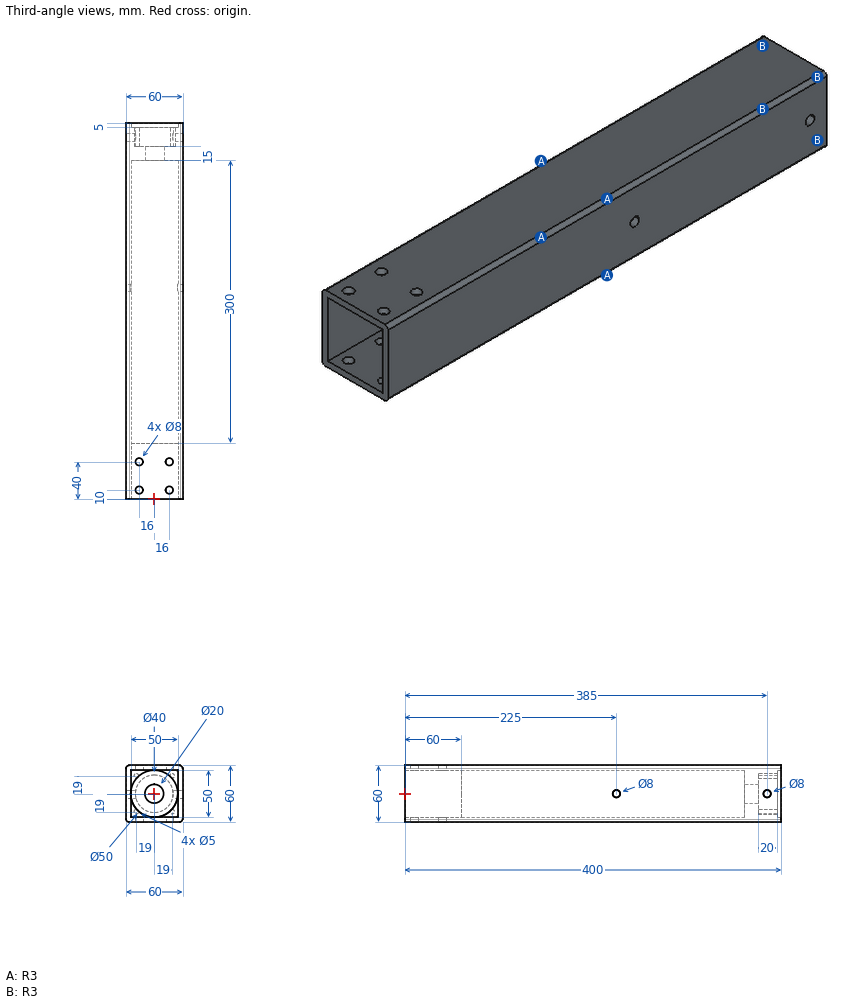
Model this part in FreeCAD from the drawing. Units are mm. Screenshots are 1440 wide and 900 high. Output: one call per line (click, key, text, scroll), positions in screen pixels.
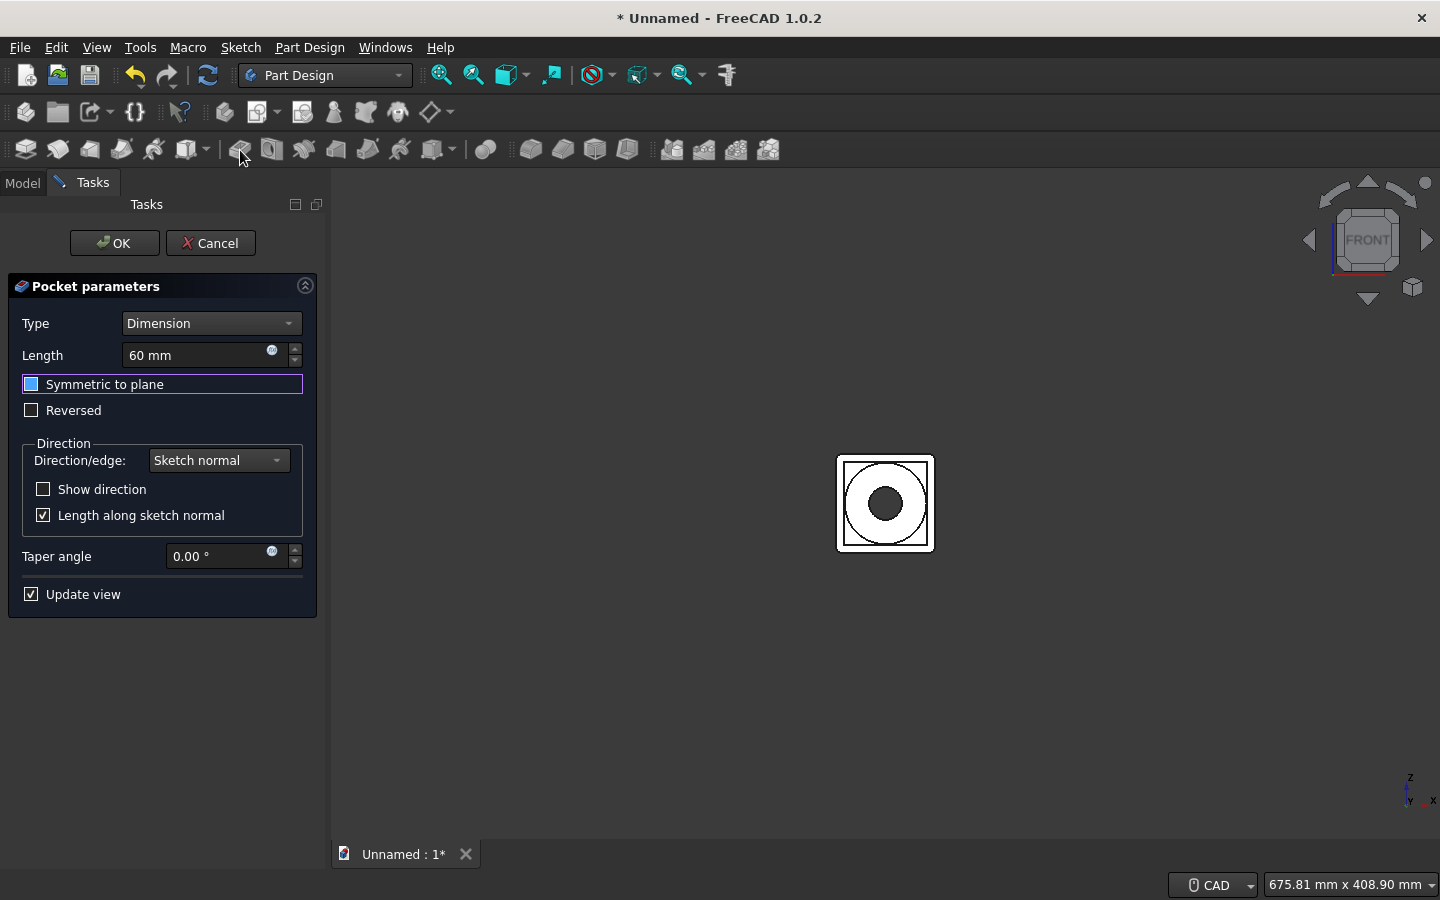
click(30, 384)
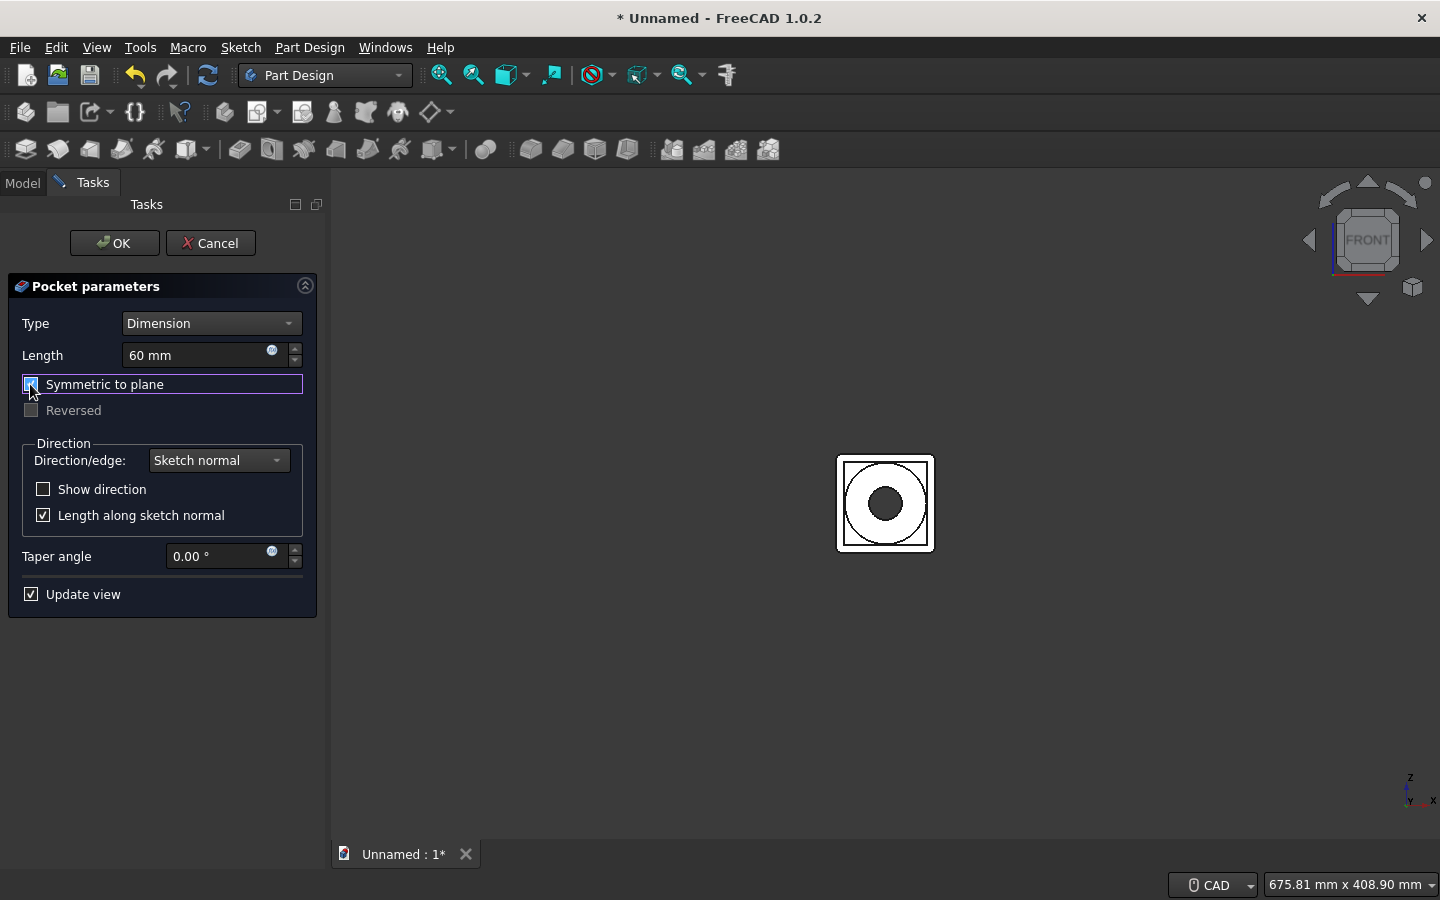
click(115, 243)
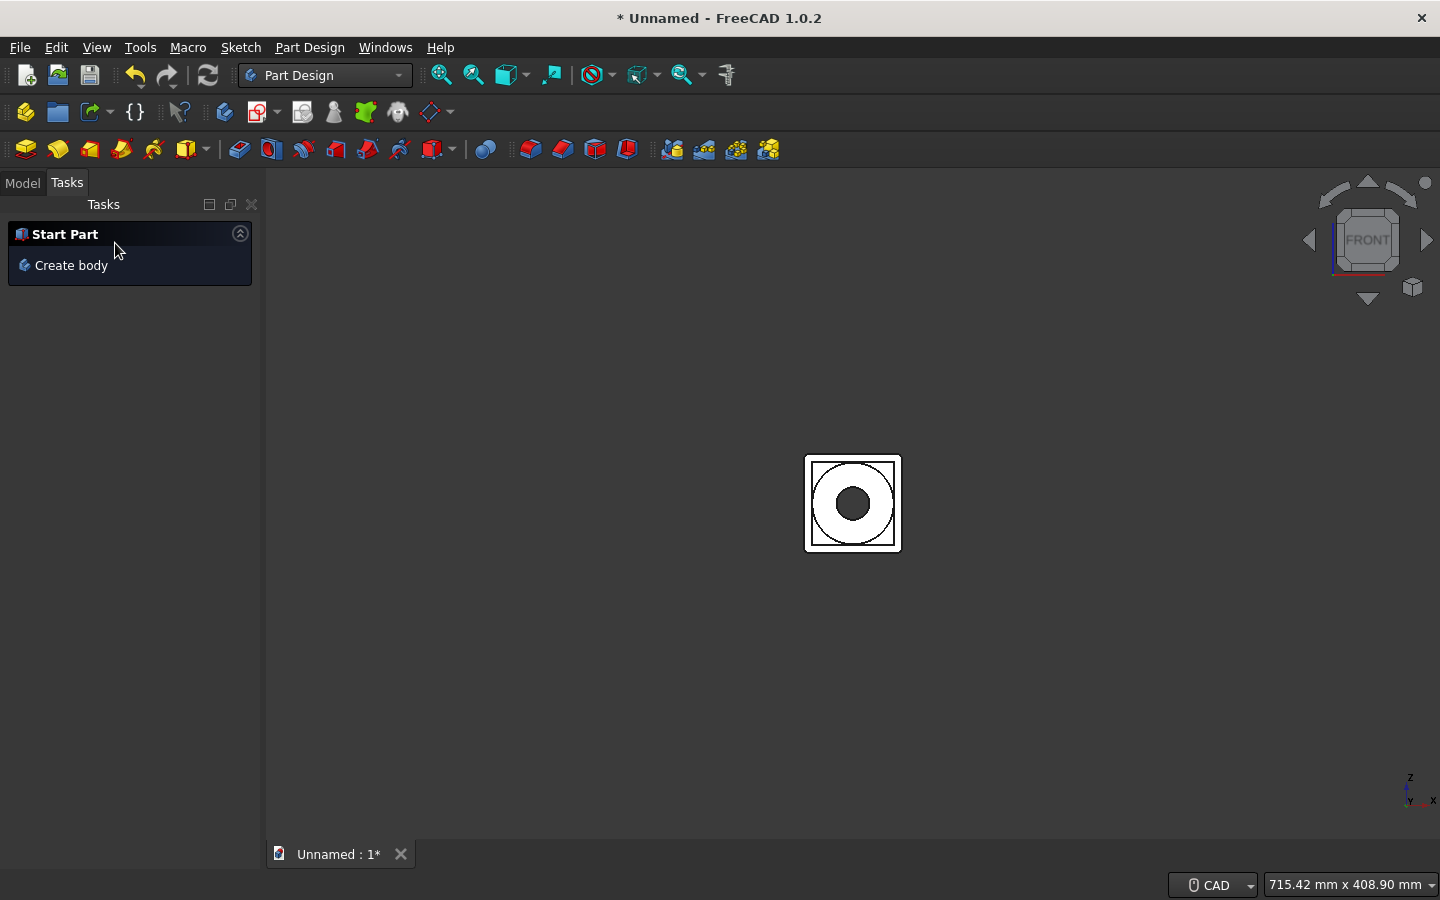
click(442, 76)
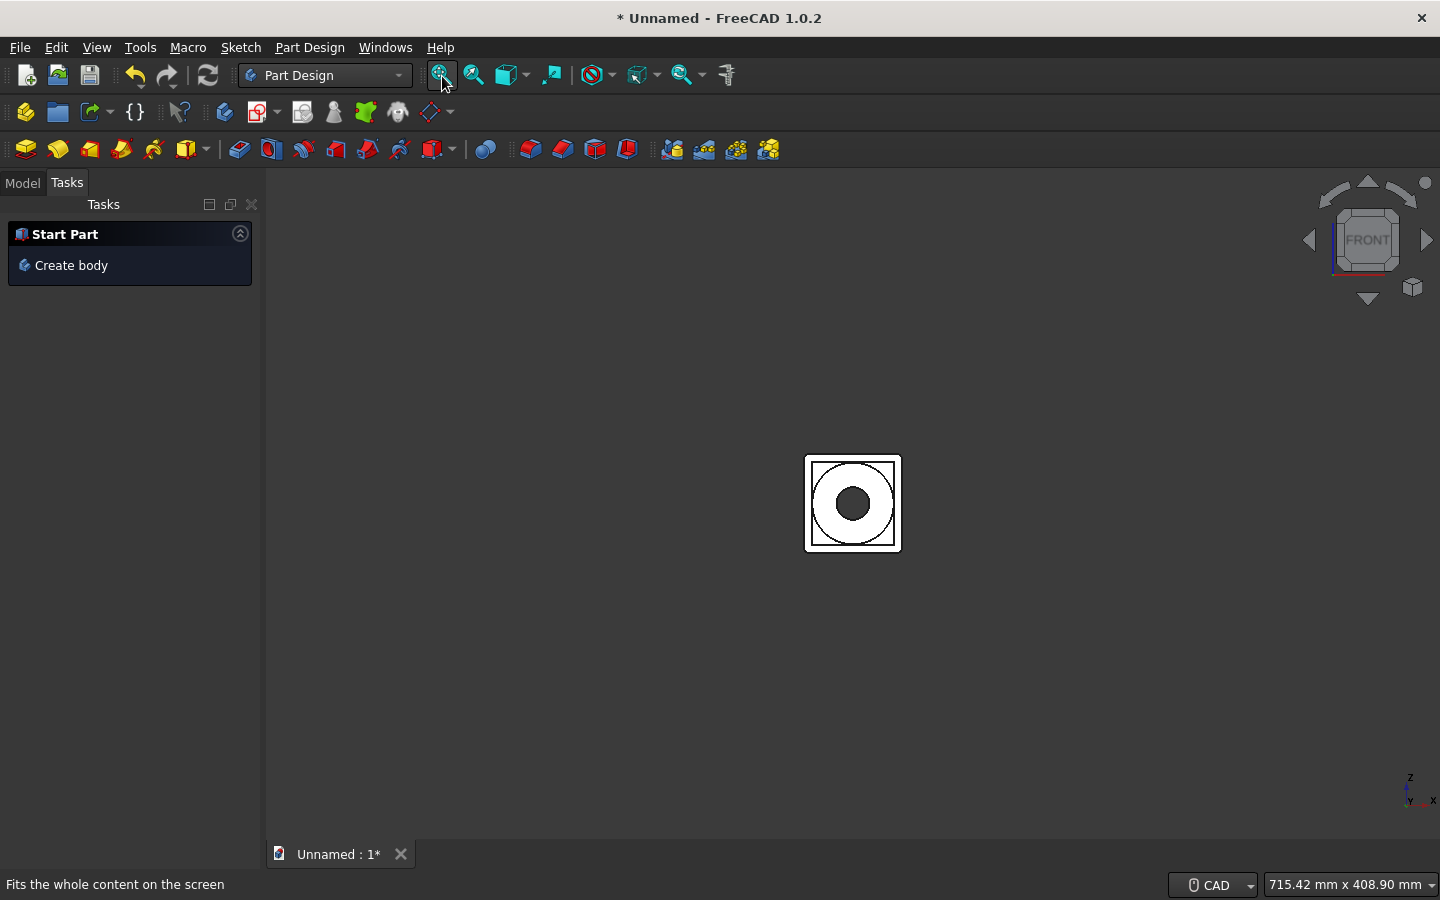
scroll(894, 544, up, 8)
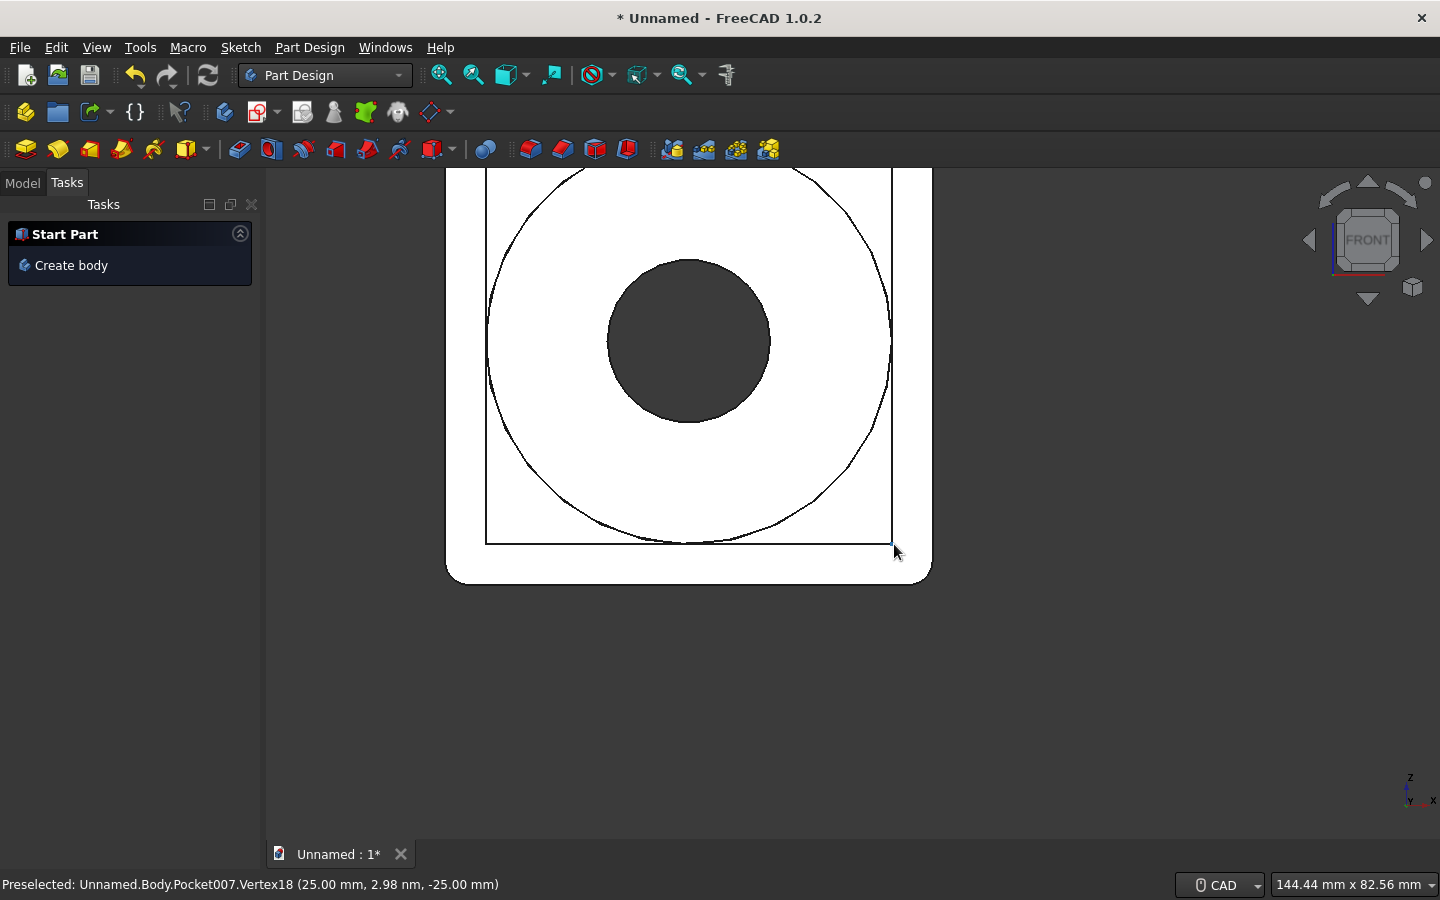
click(442, 76)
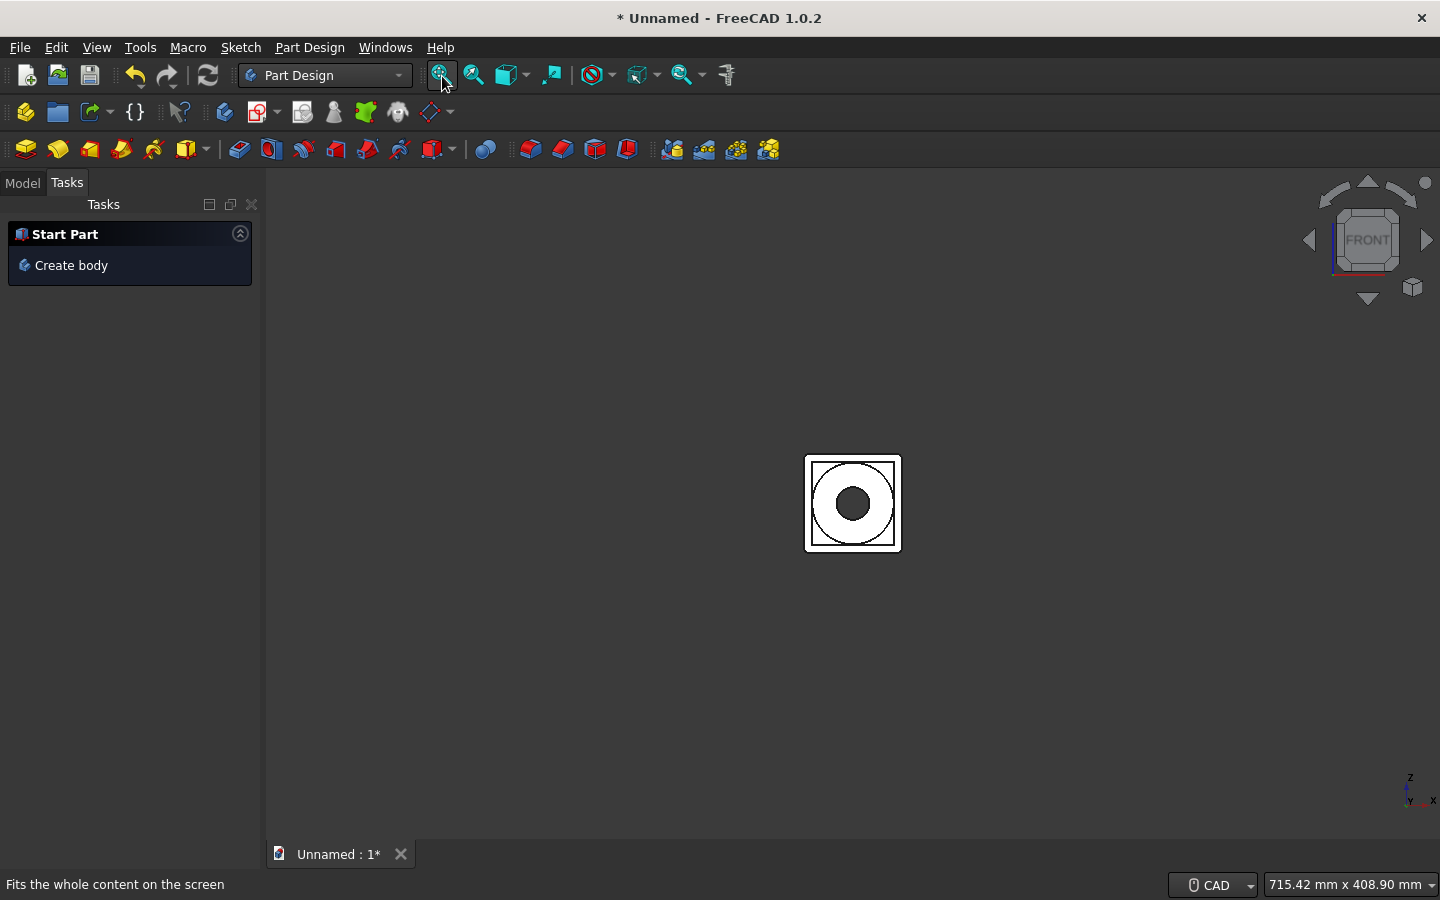
key(0)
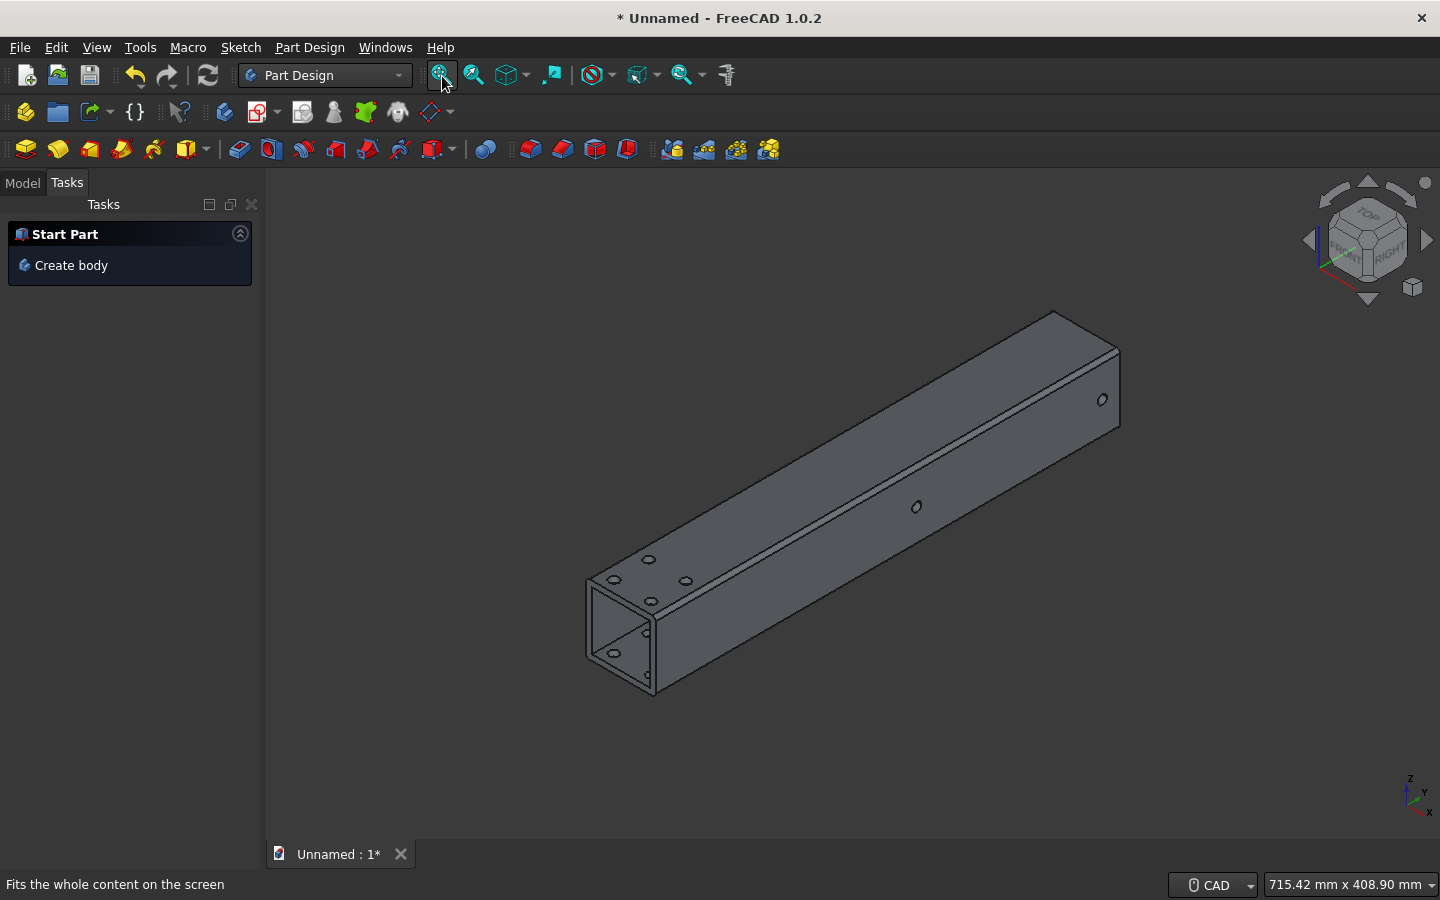
scroll(1111, 420, up, 8)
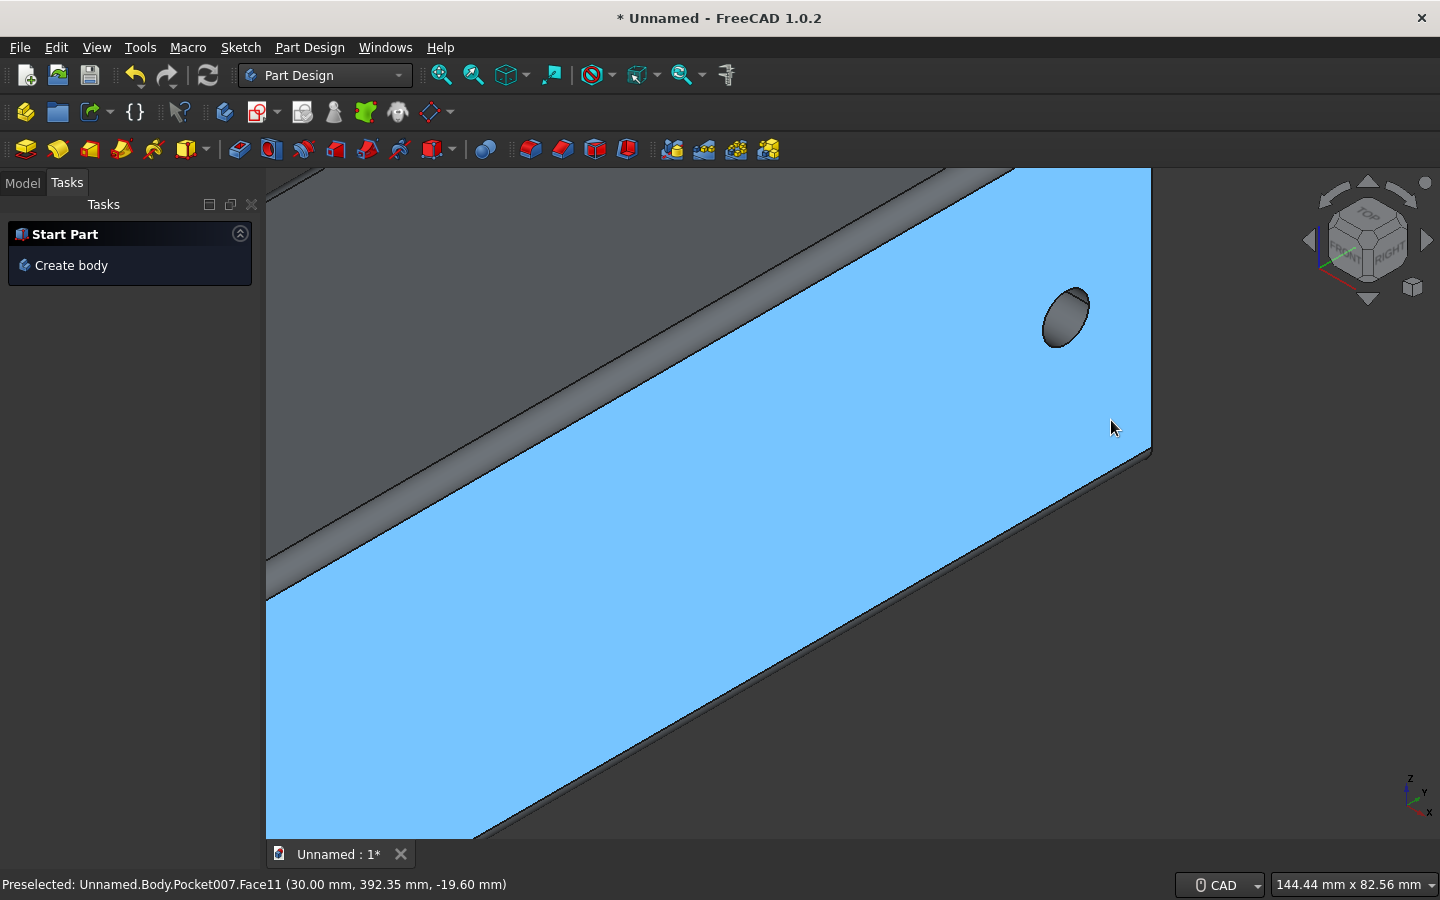
click(442, 76)